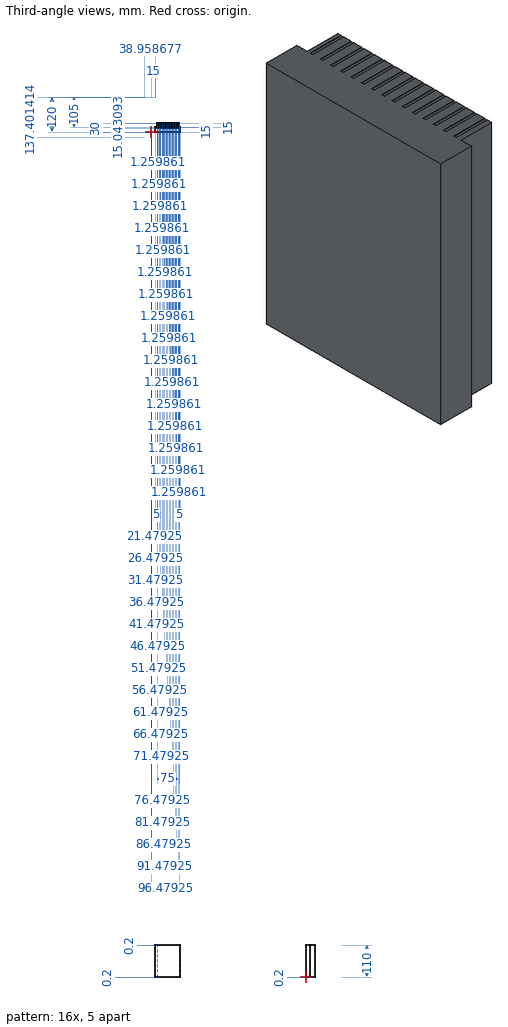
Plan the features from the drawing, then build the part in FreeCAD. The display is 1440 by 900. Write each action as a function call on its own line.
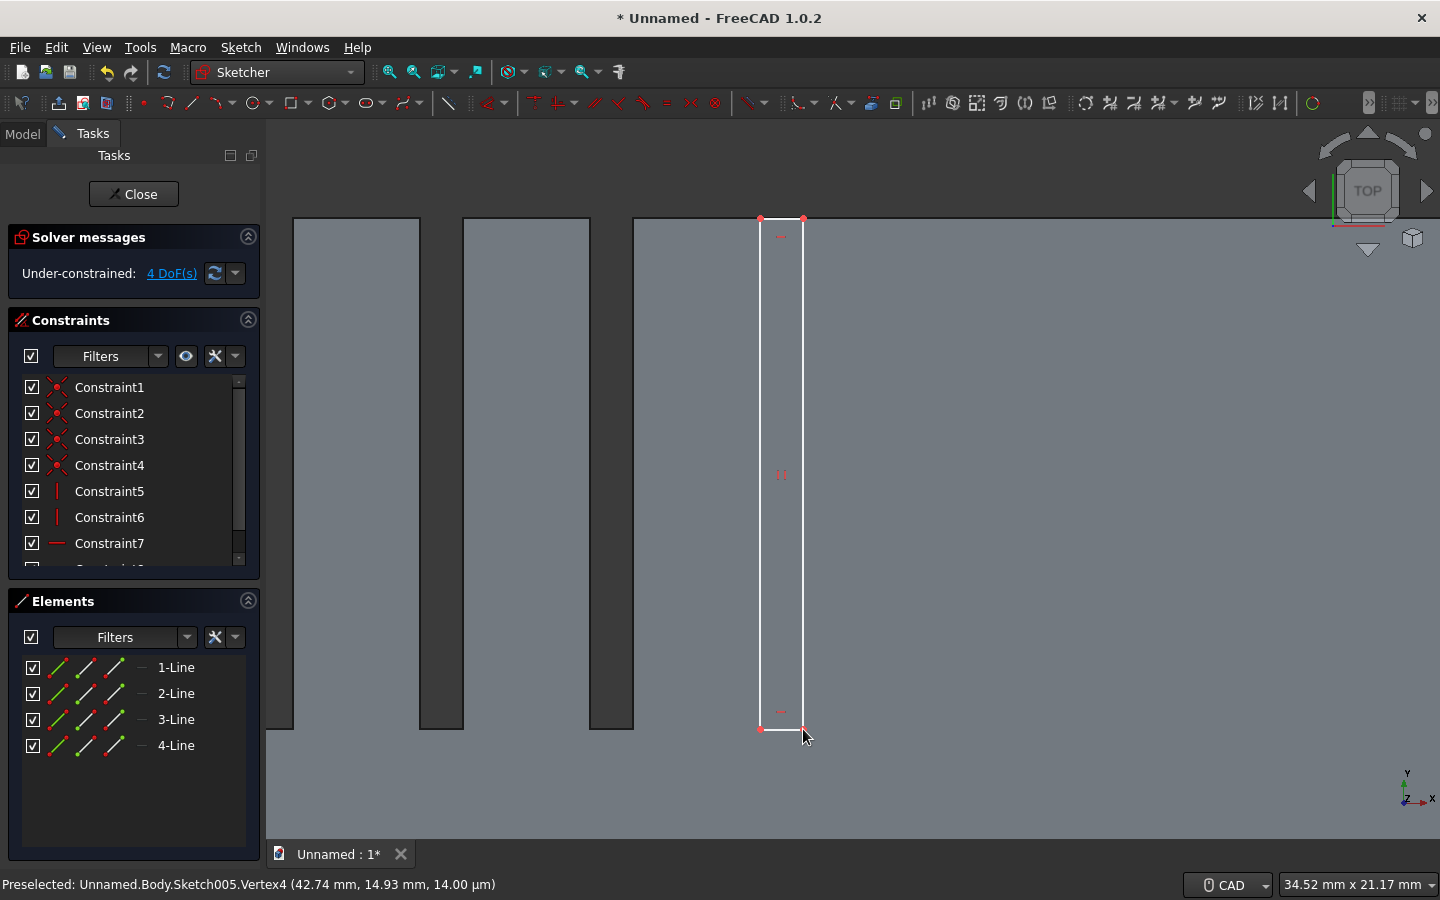
click(488, 104)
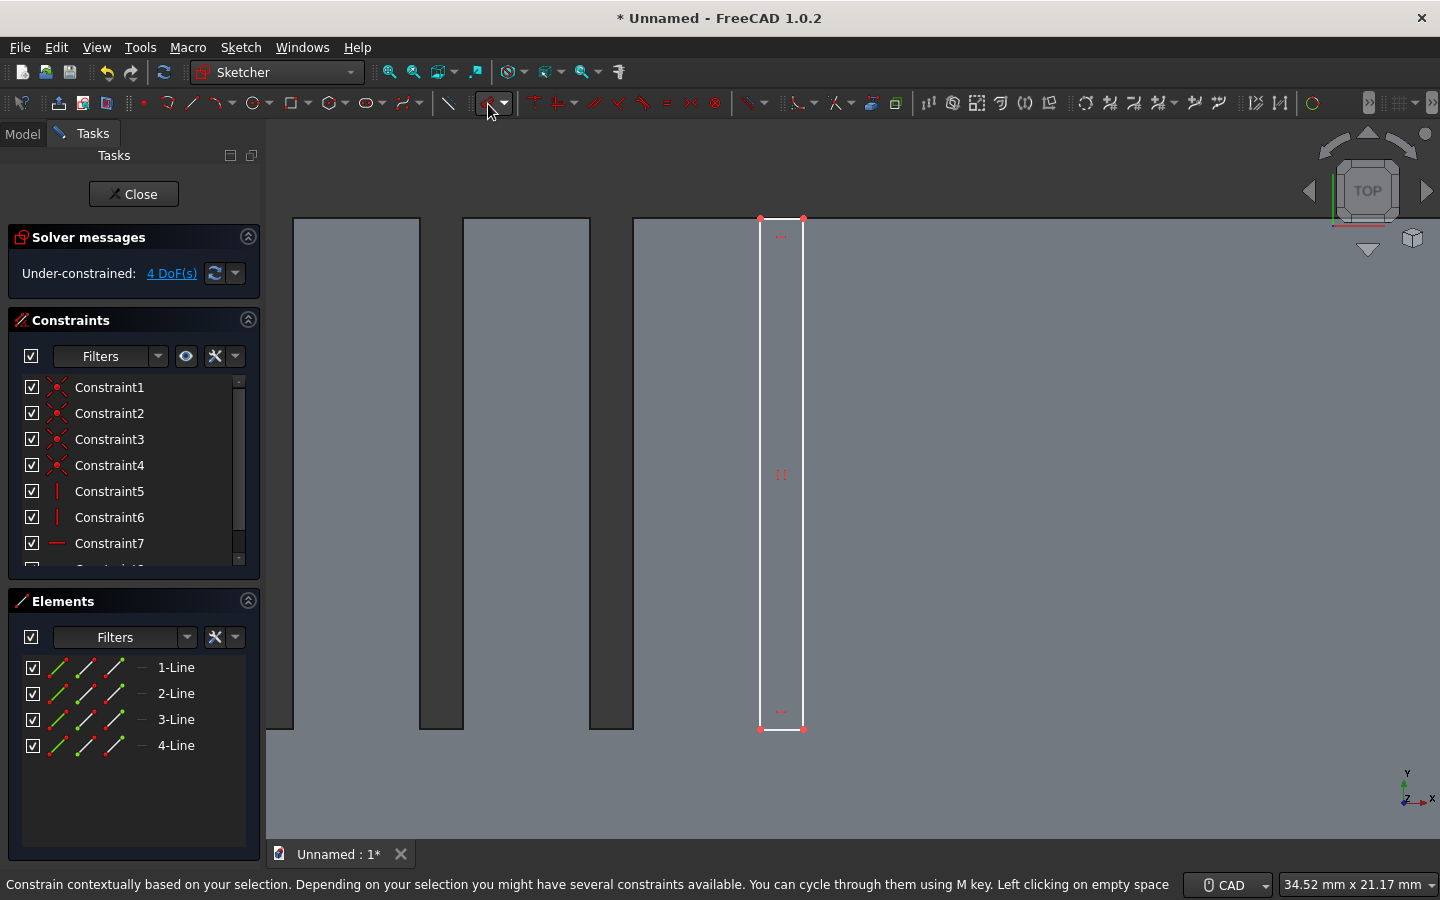
click(760, 219)
click(818, 515)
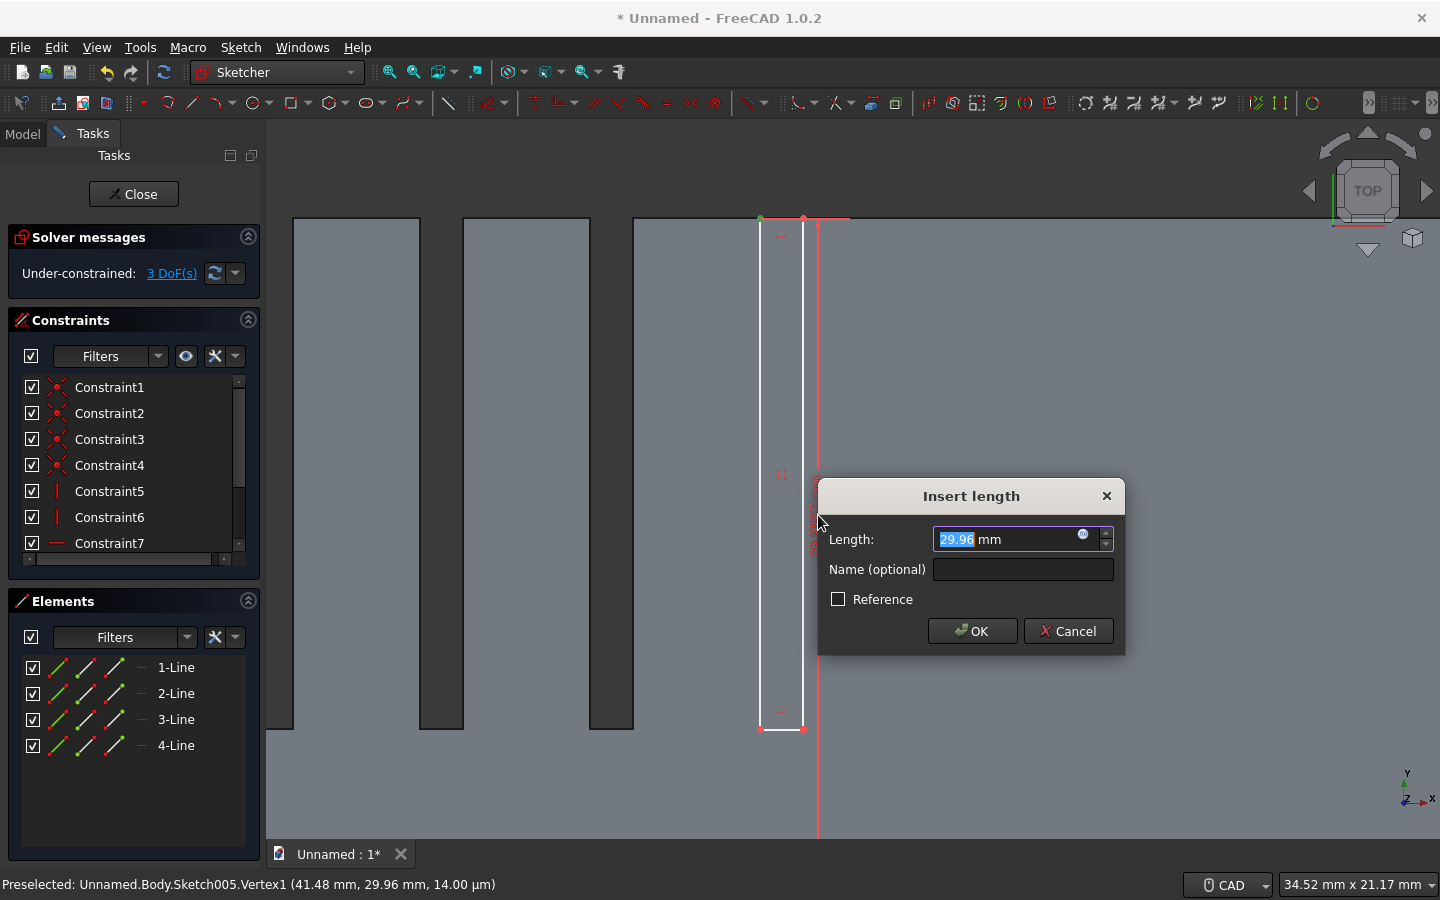
text(30)
key(Return)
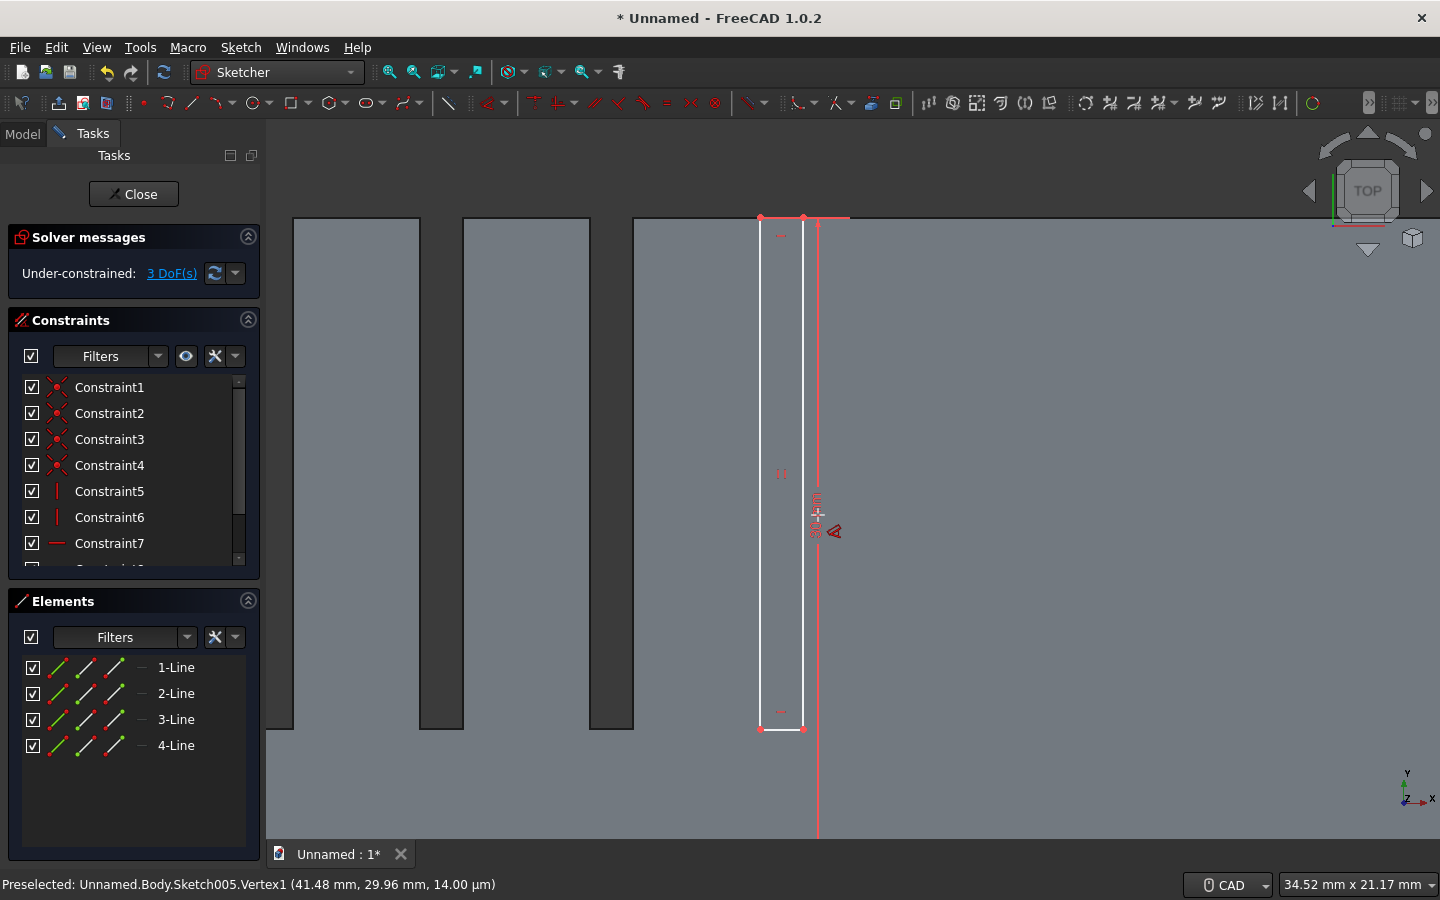
click(773, 730)
click(782, 764)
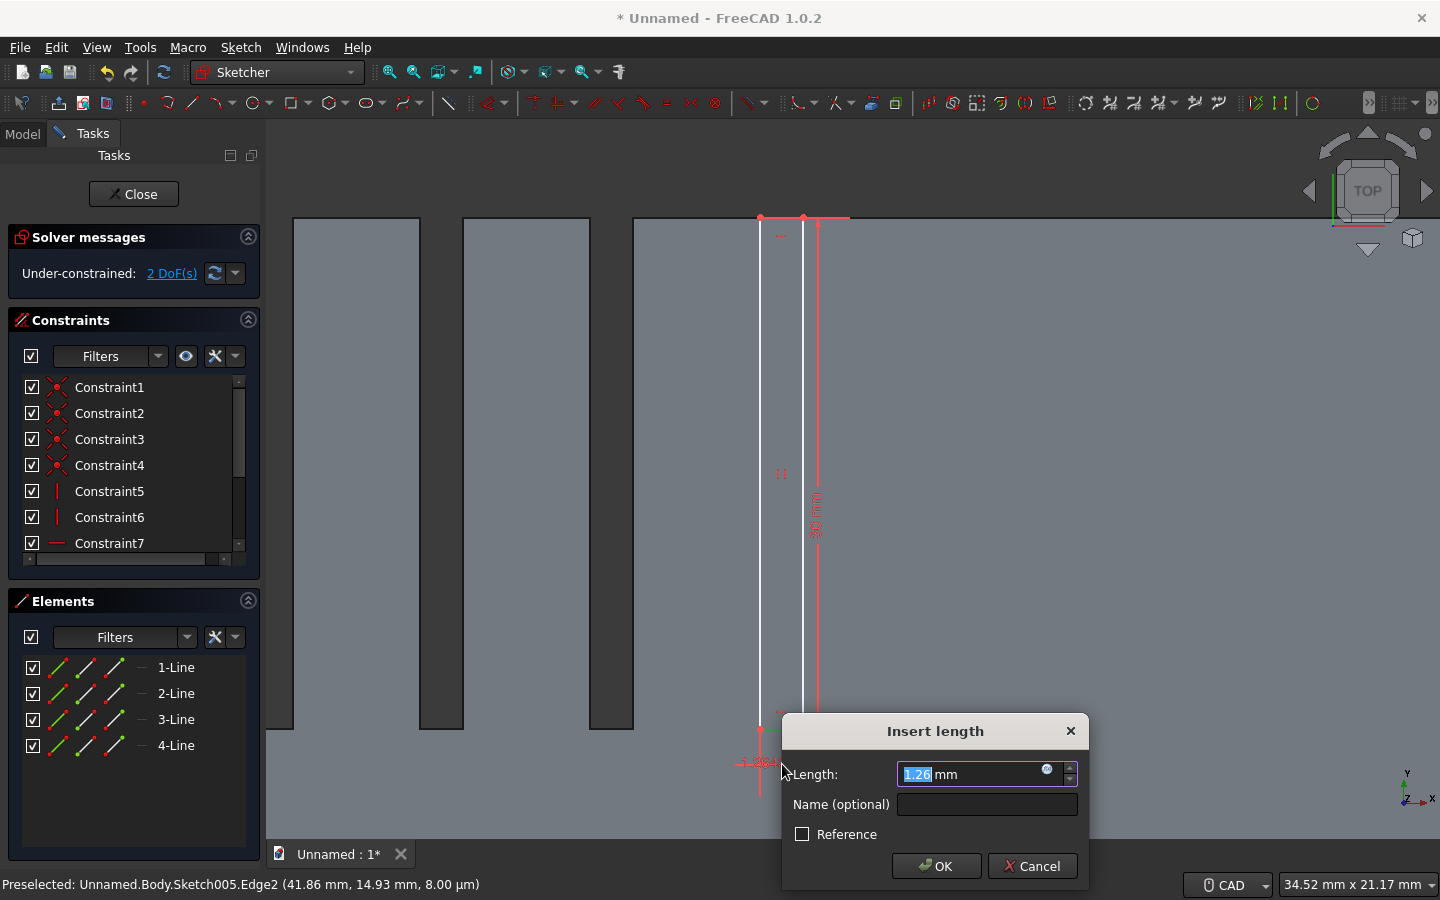
text(1.259861)
key(Return)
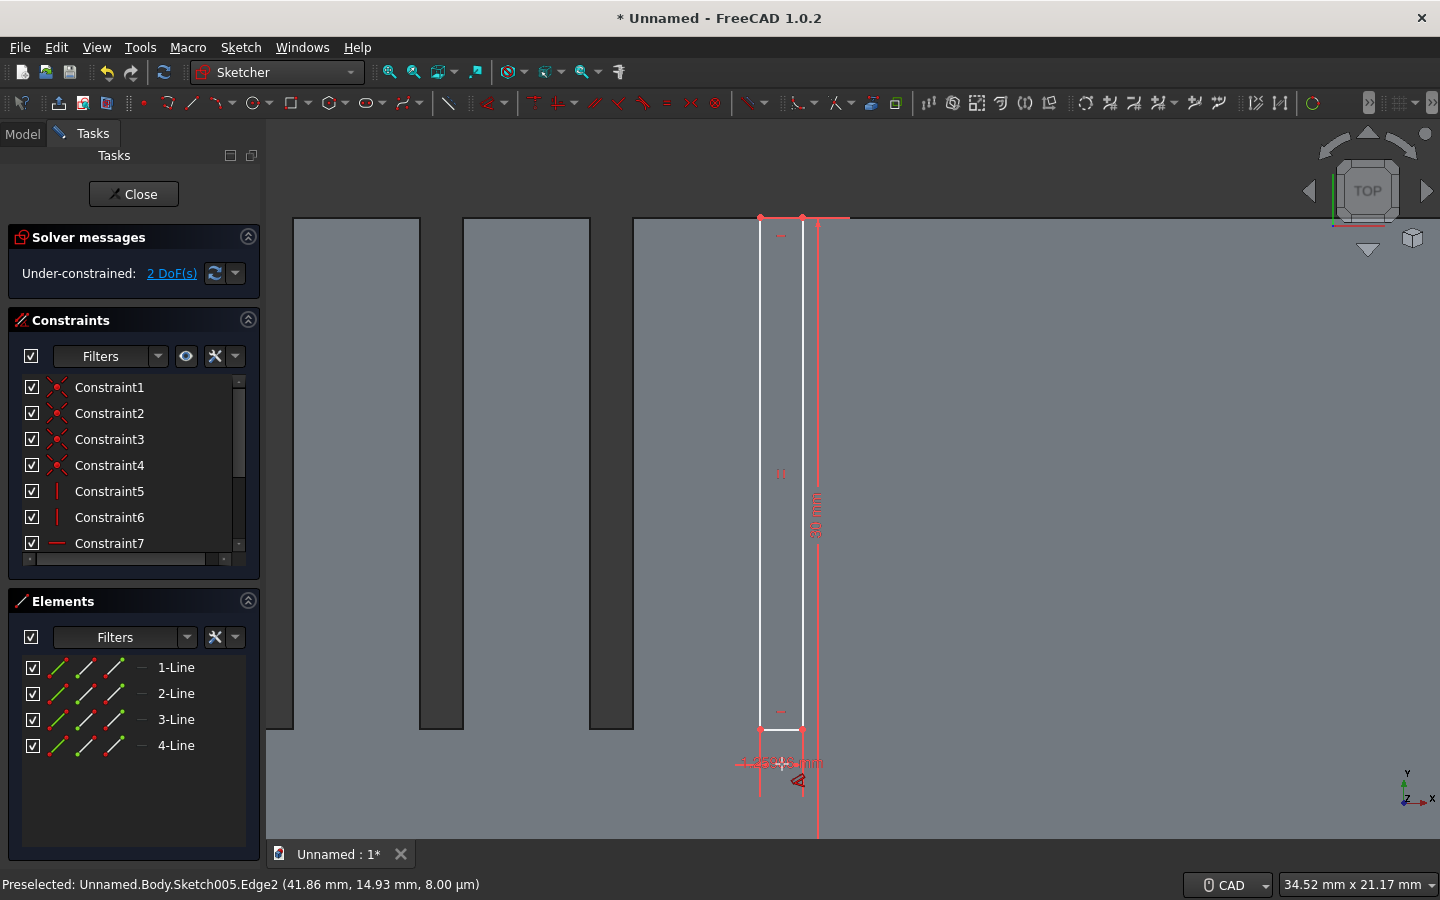
click(760, 371)
click(726, 474)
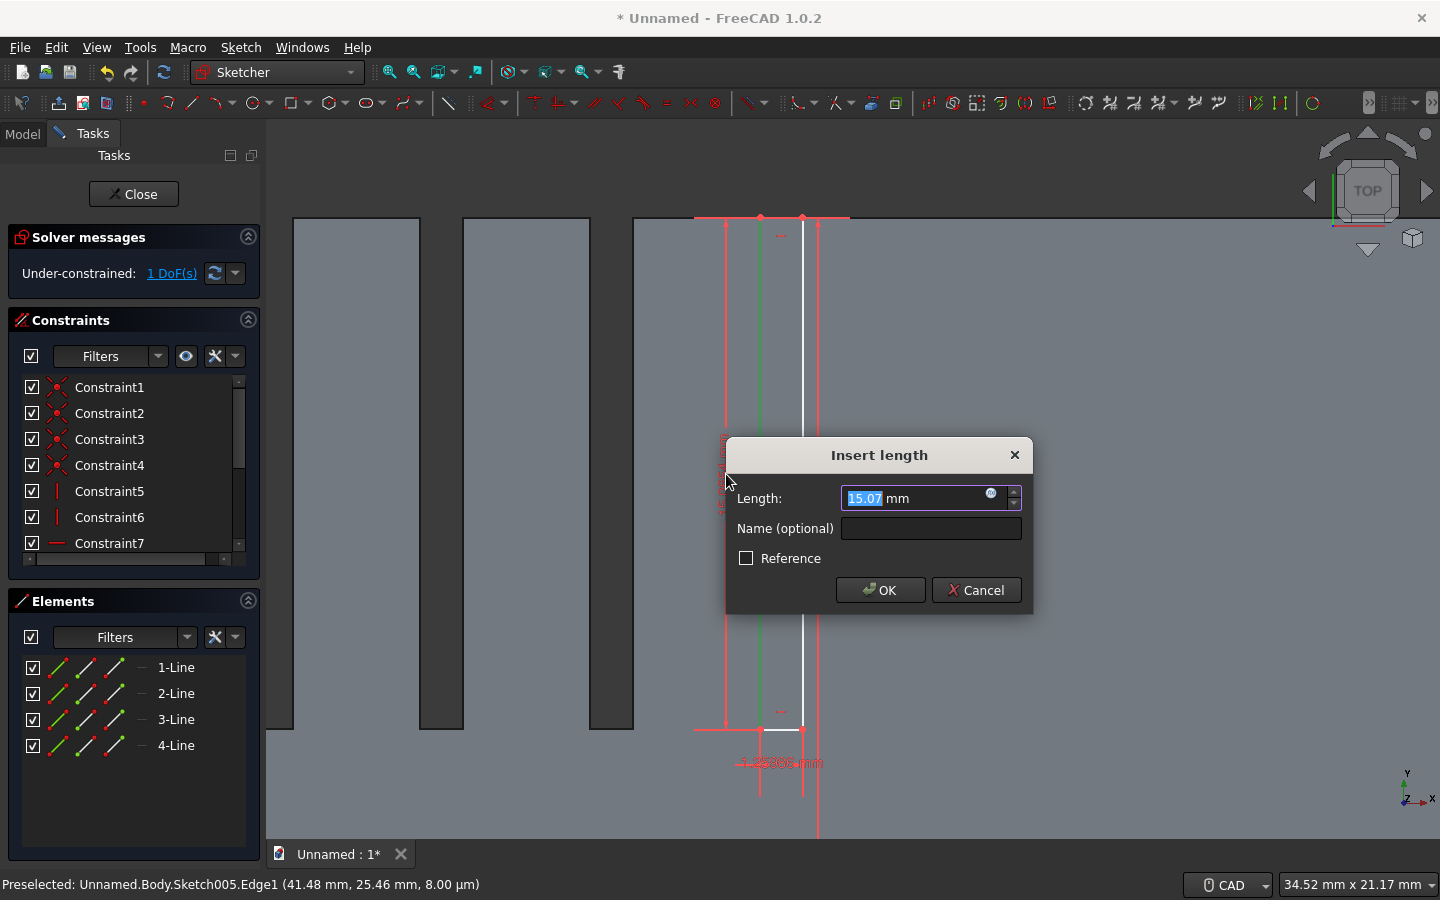
text(15.043093)
key(Return)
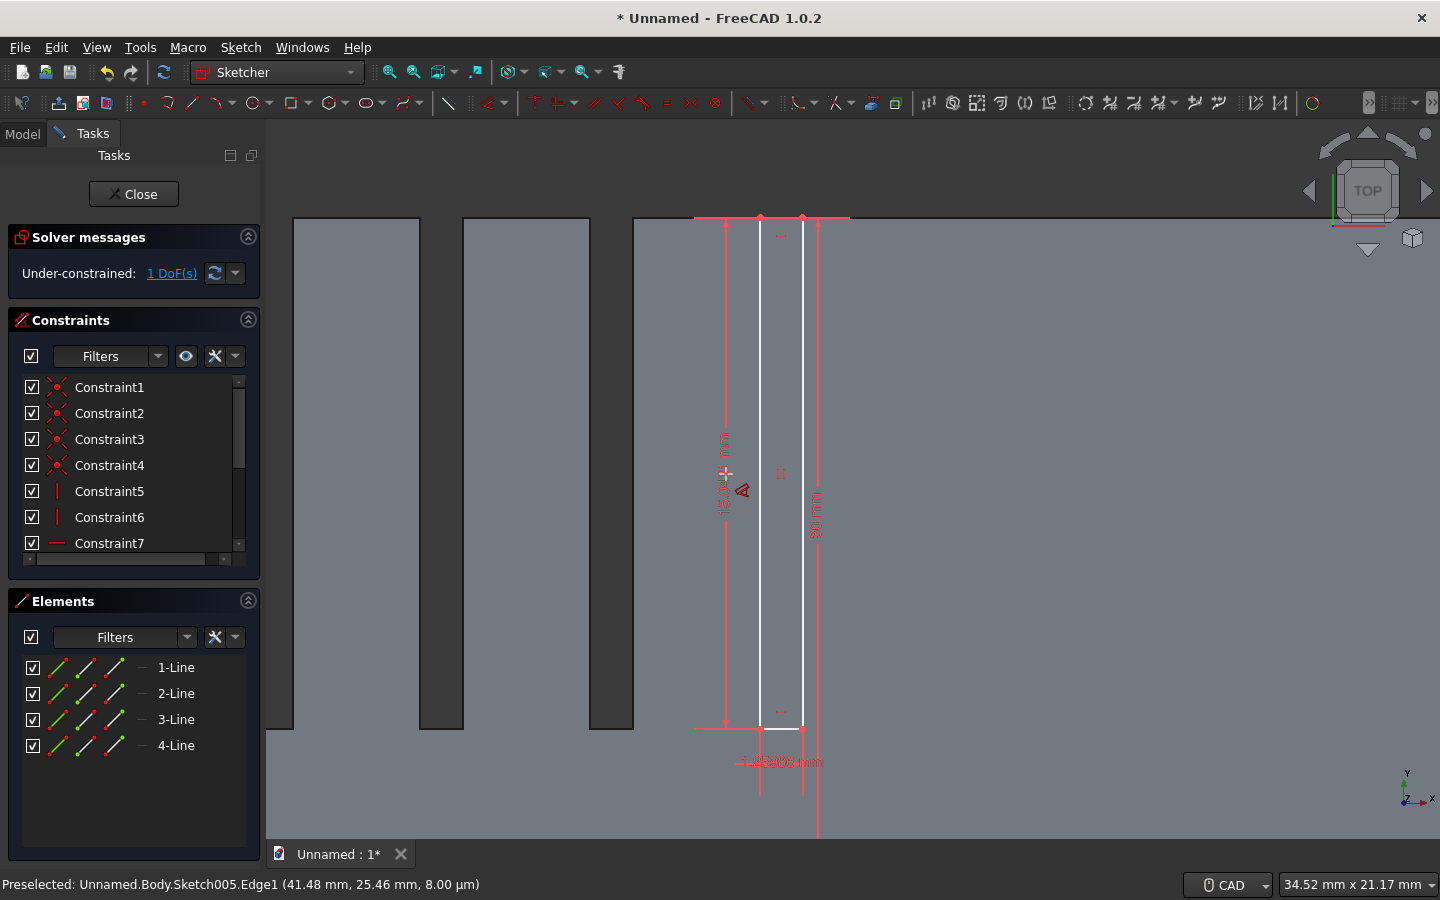
click(760, 218)
click(527, 184)